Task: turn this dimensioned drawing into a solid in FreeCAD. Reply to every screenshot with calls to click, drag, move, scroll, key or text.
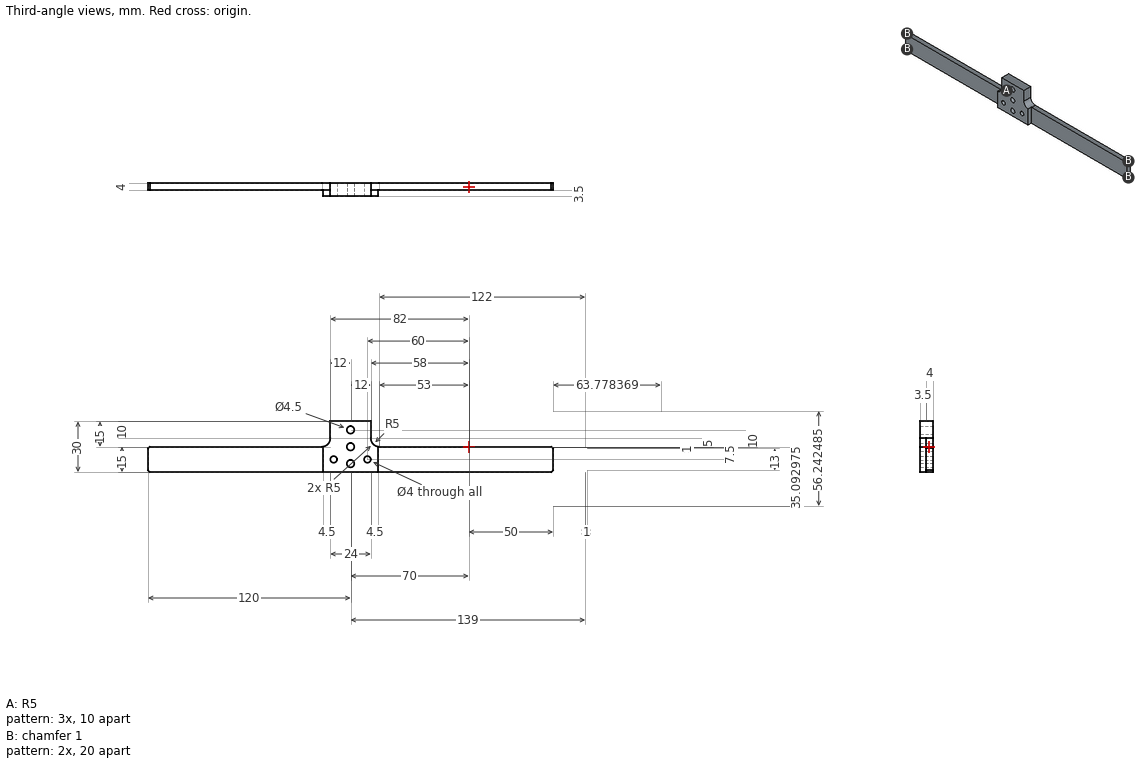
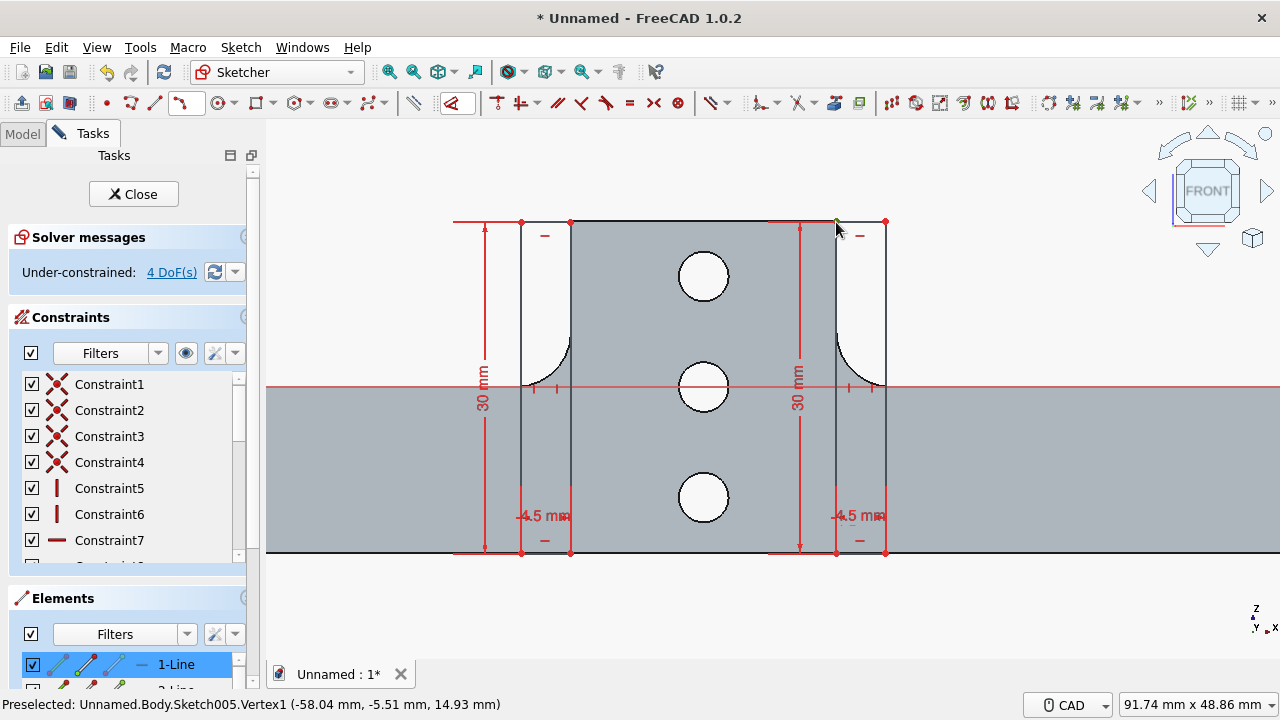
key(l)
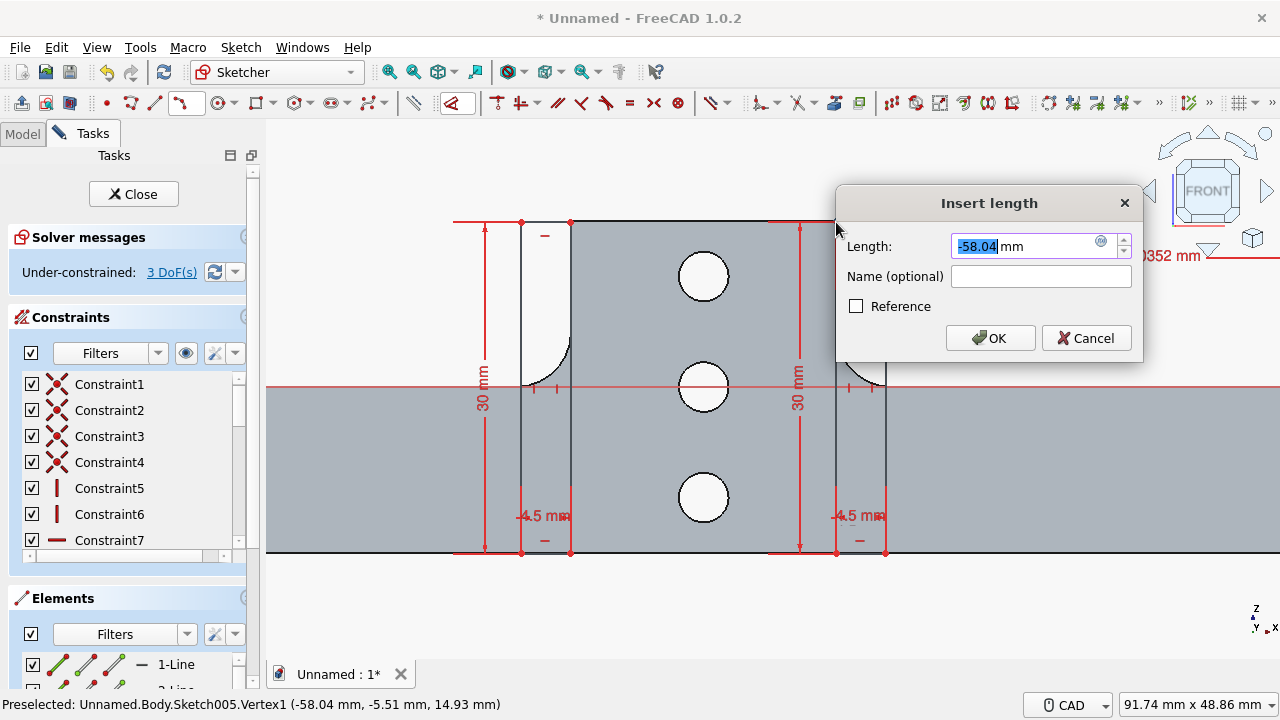
text(-58)
key(Return)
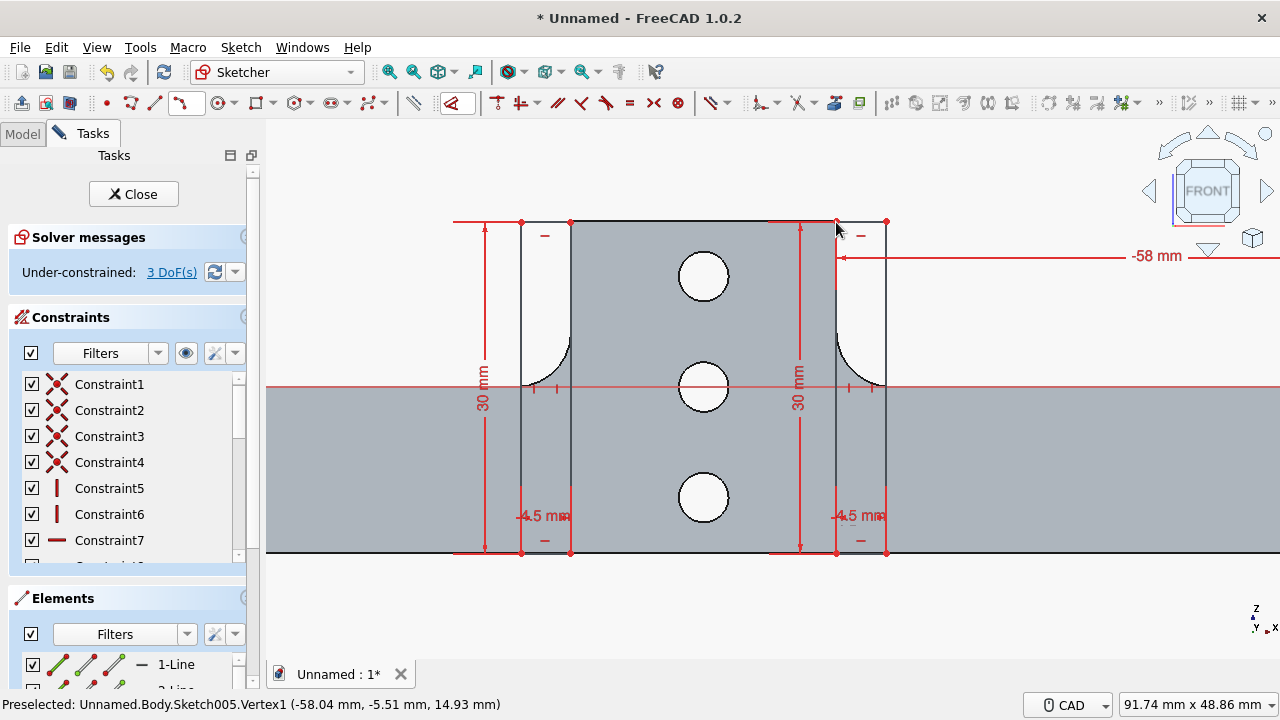
click(836, 222)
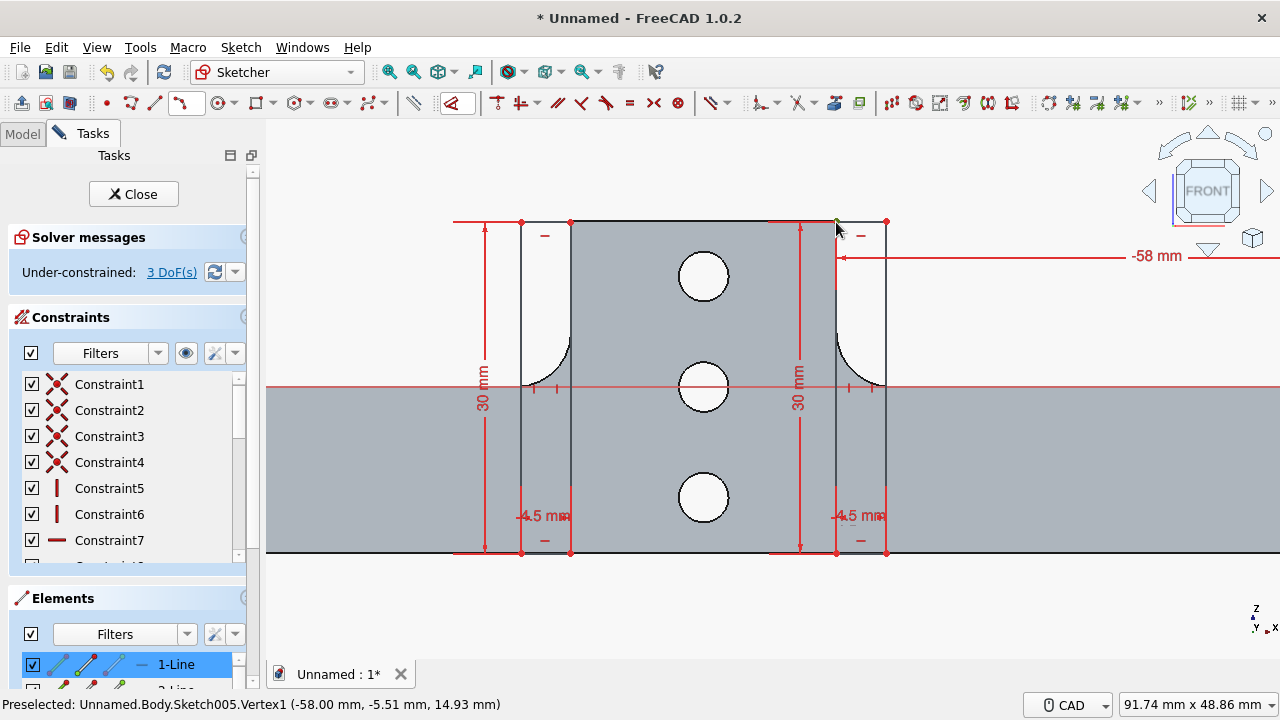
key(i)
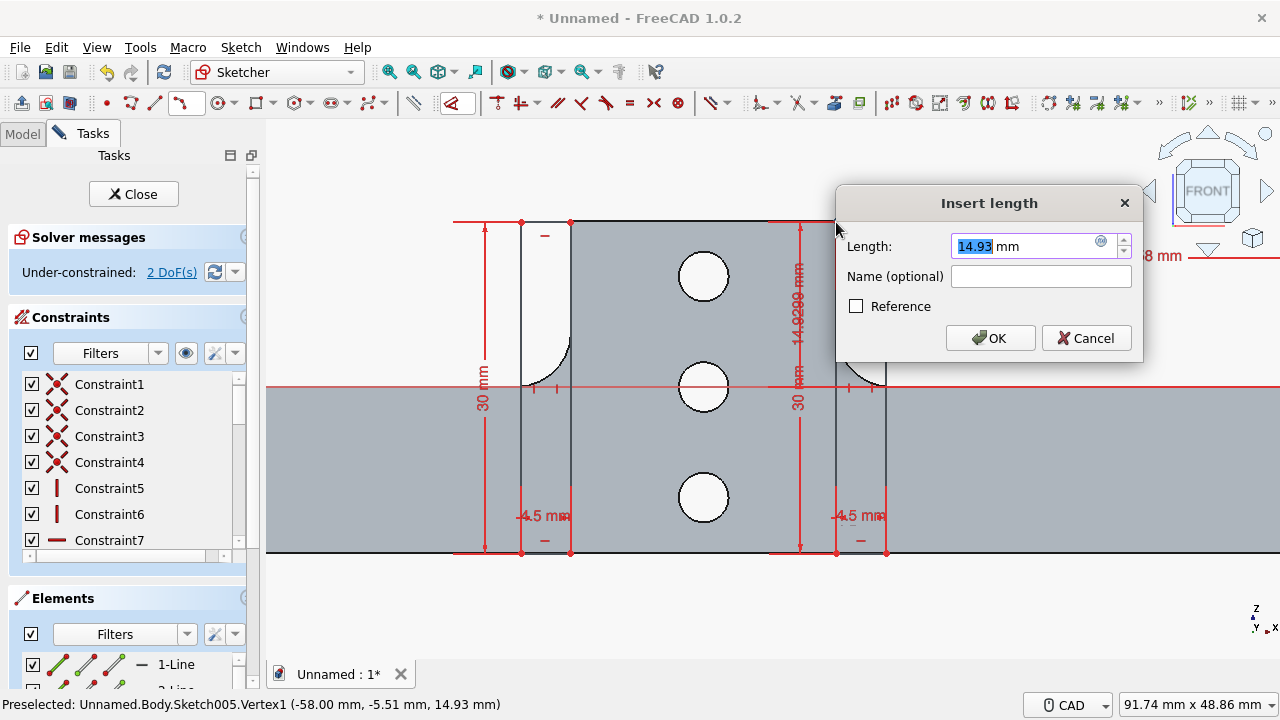
text(15)
key(Return)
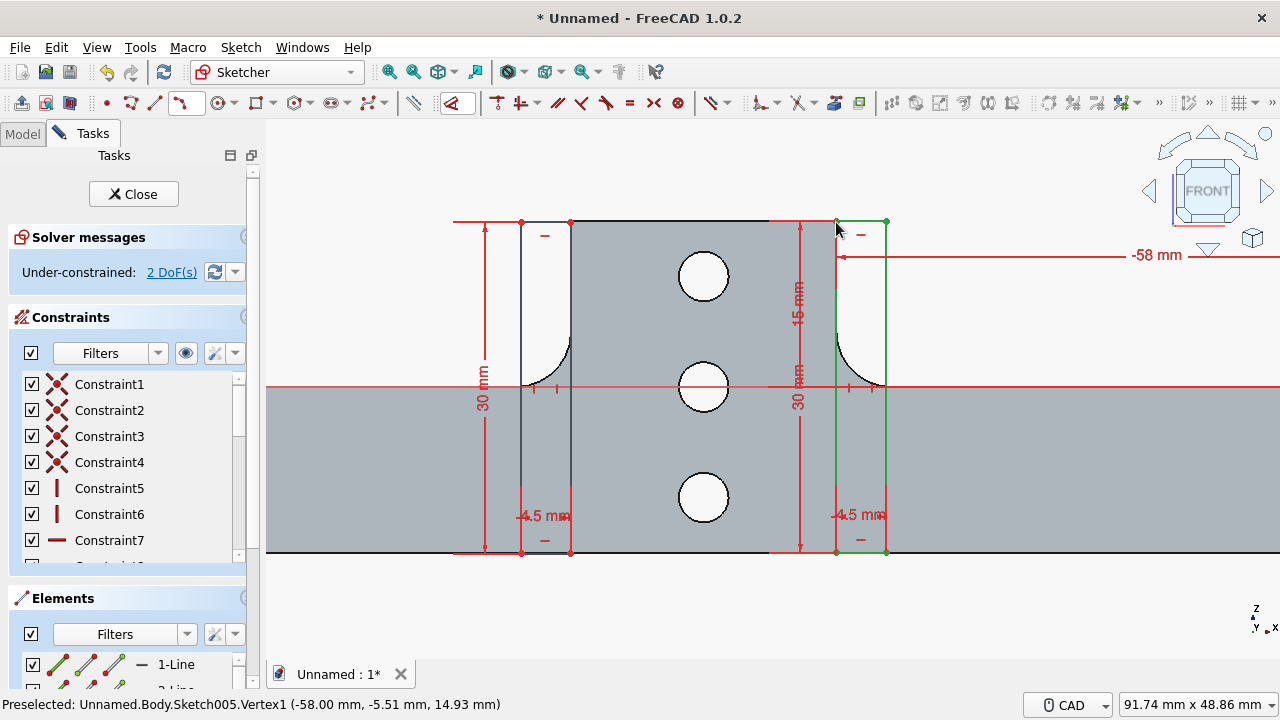
click(521, 222)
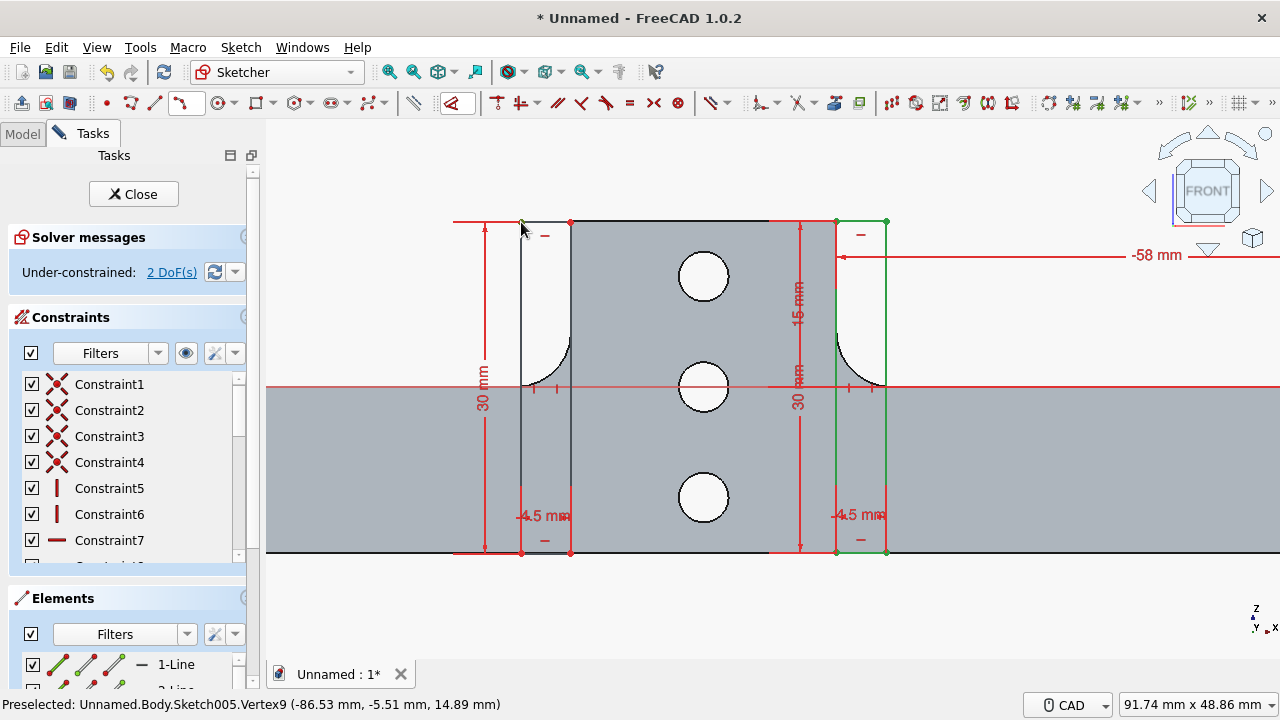
key(i)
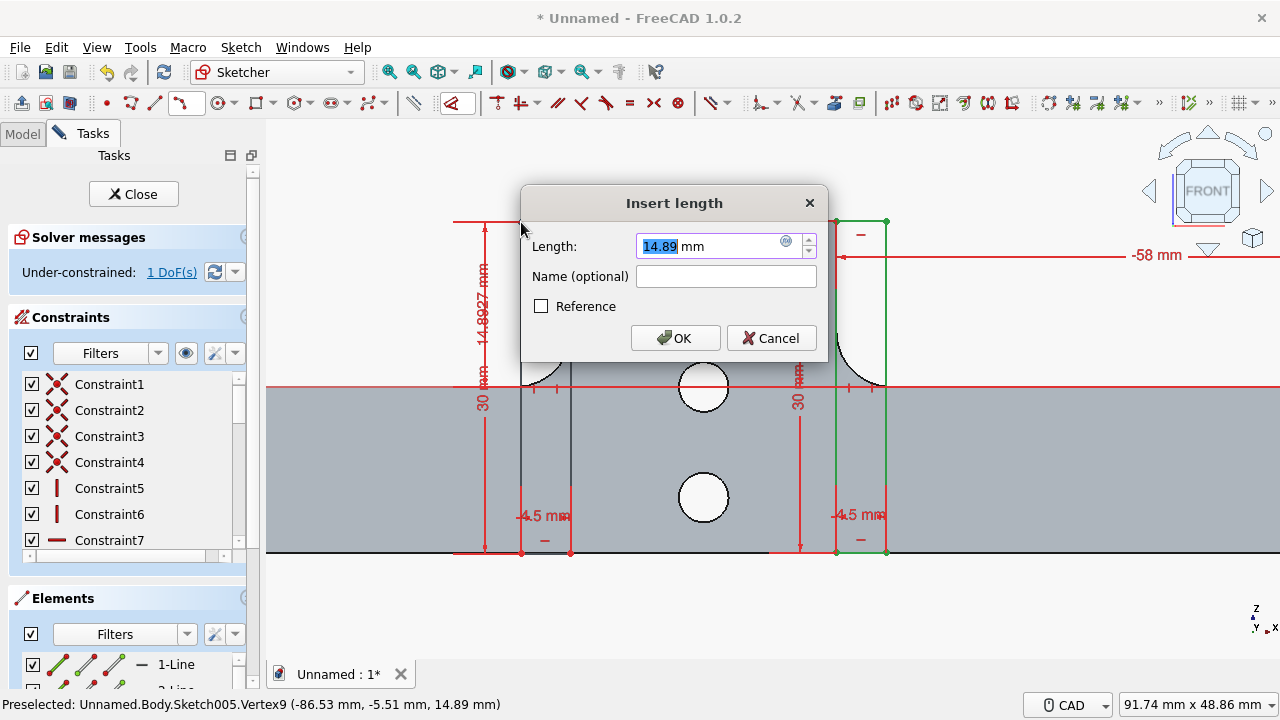
text(15)
key(Return)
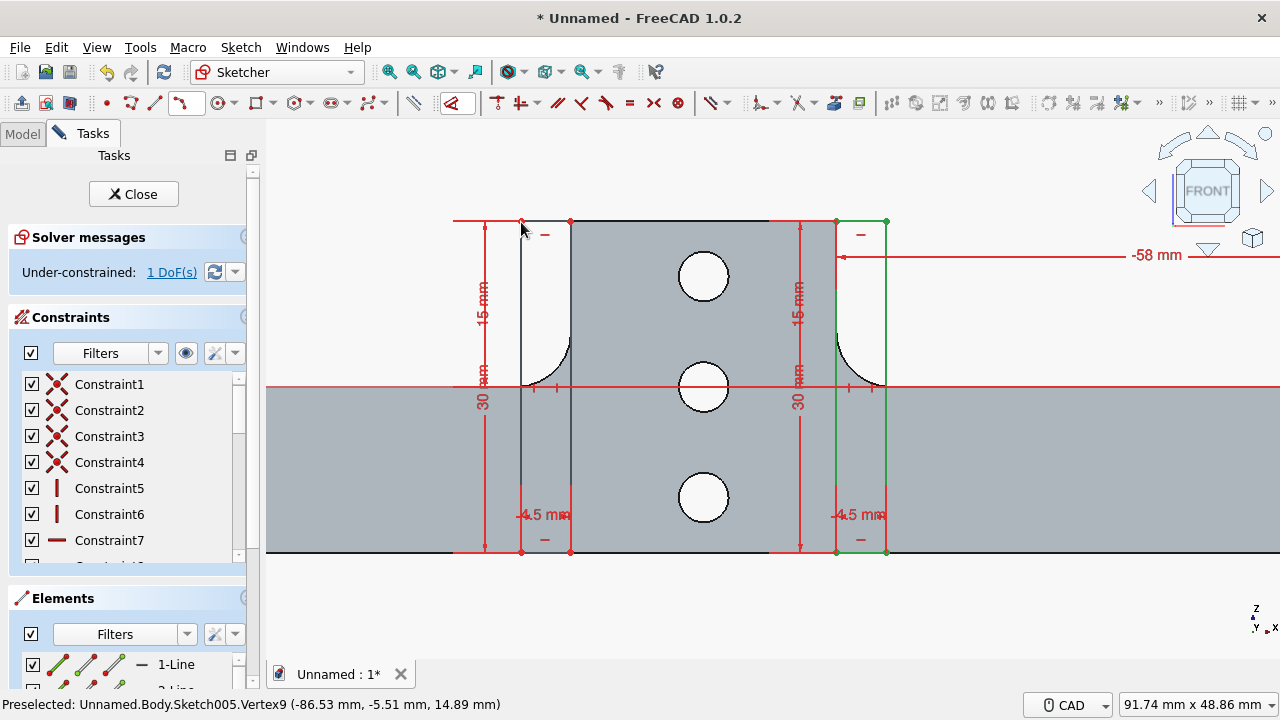
click(571, 553)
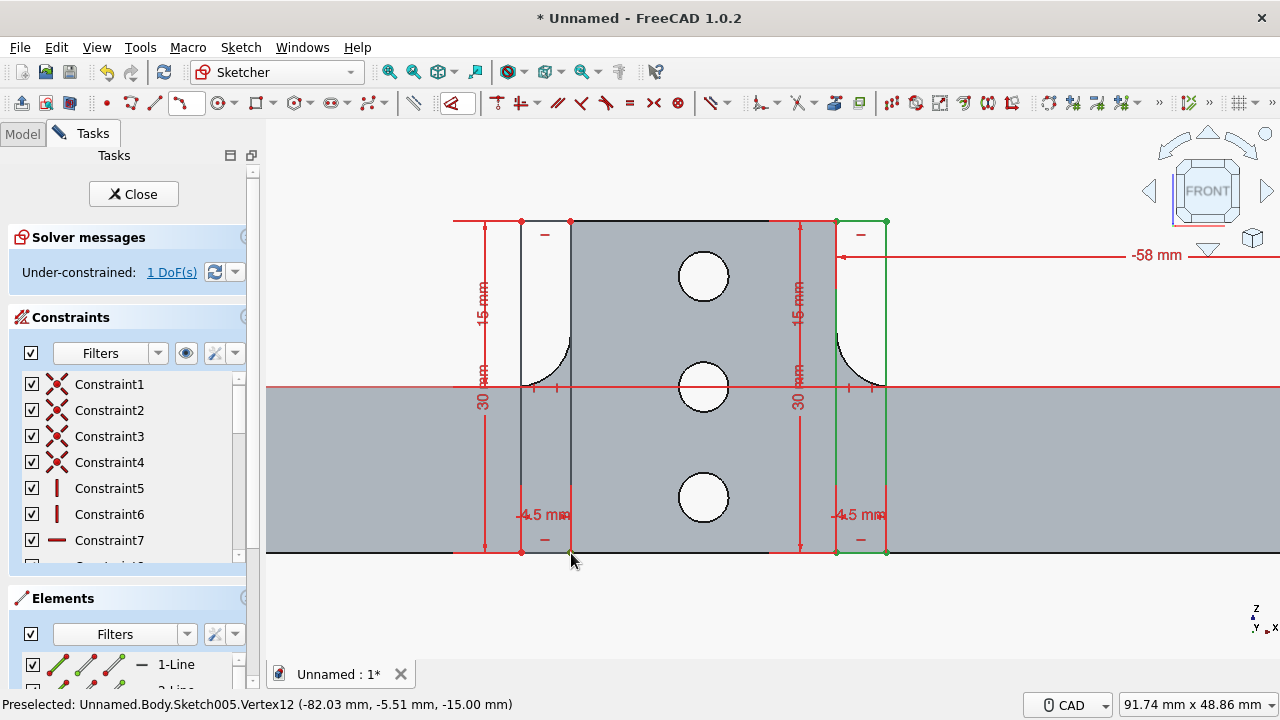
key(l)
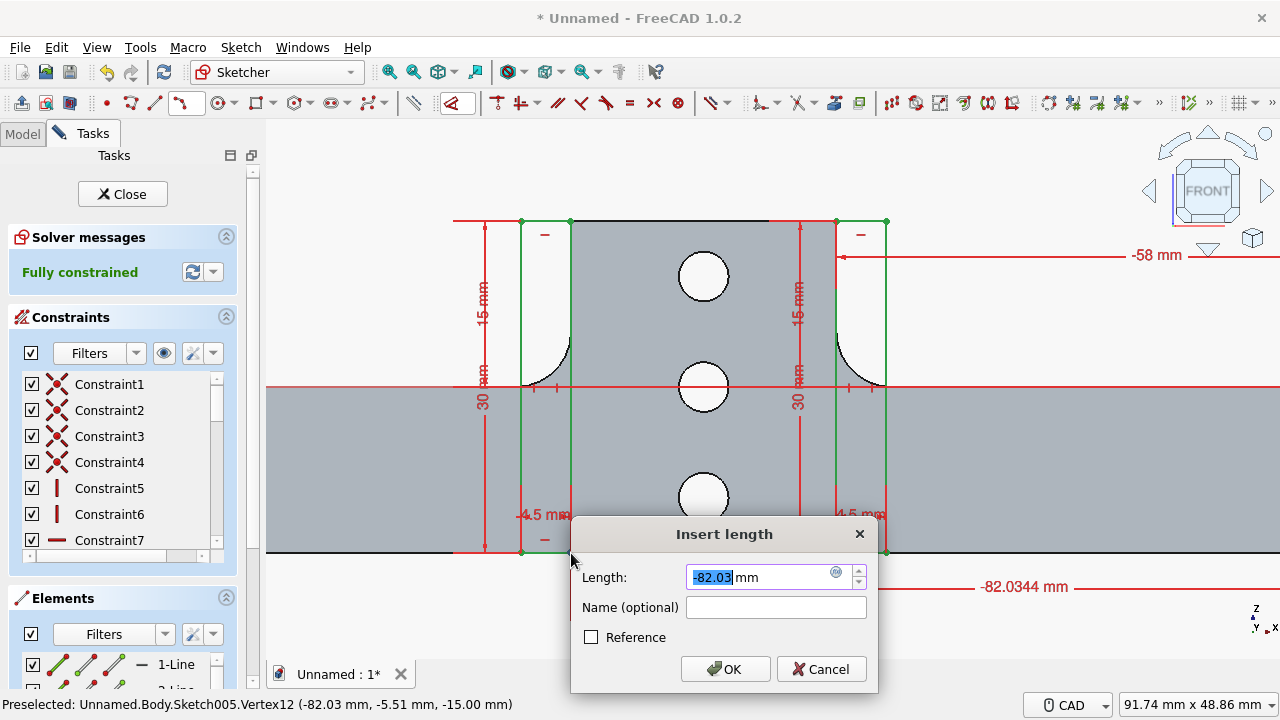
text(-82)
key(Return)